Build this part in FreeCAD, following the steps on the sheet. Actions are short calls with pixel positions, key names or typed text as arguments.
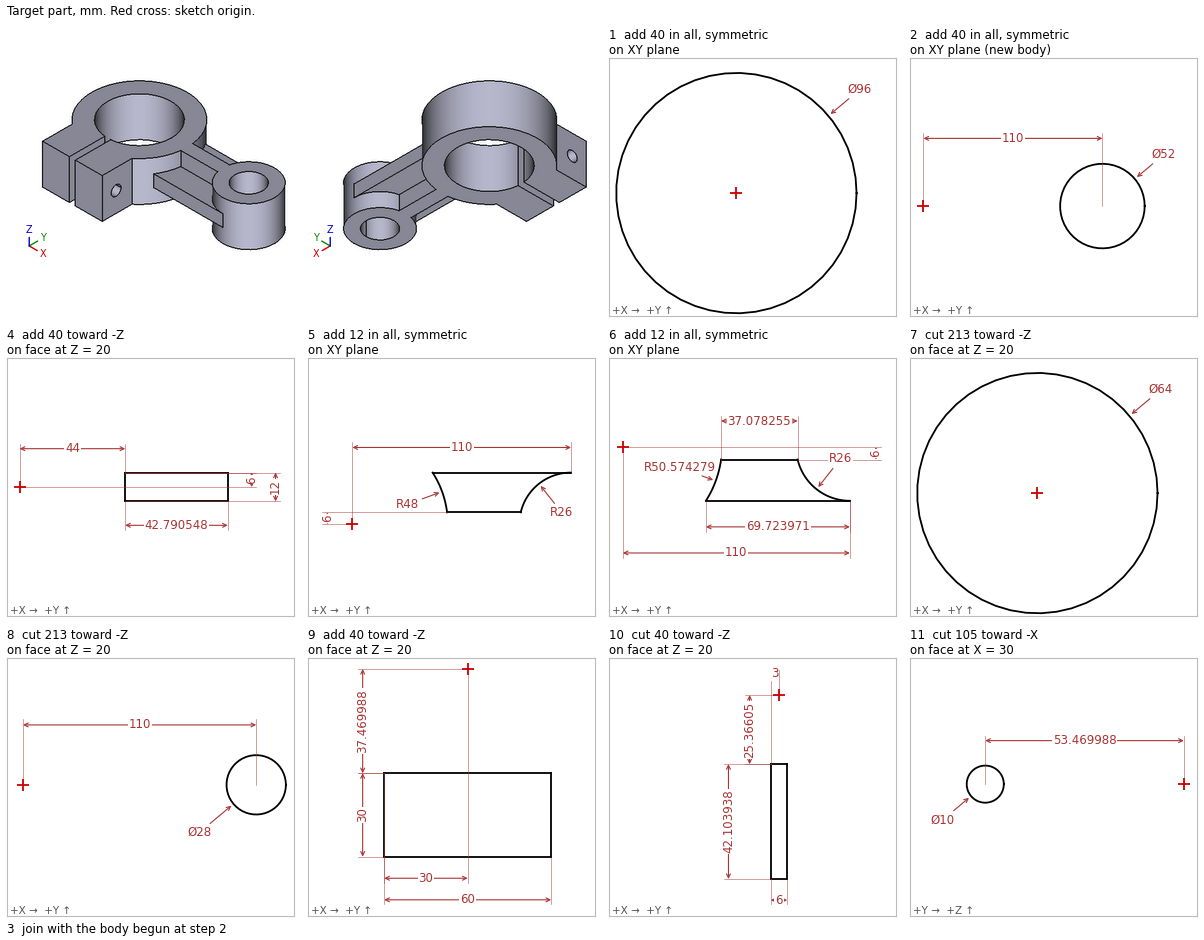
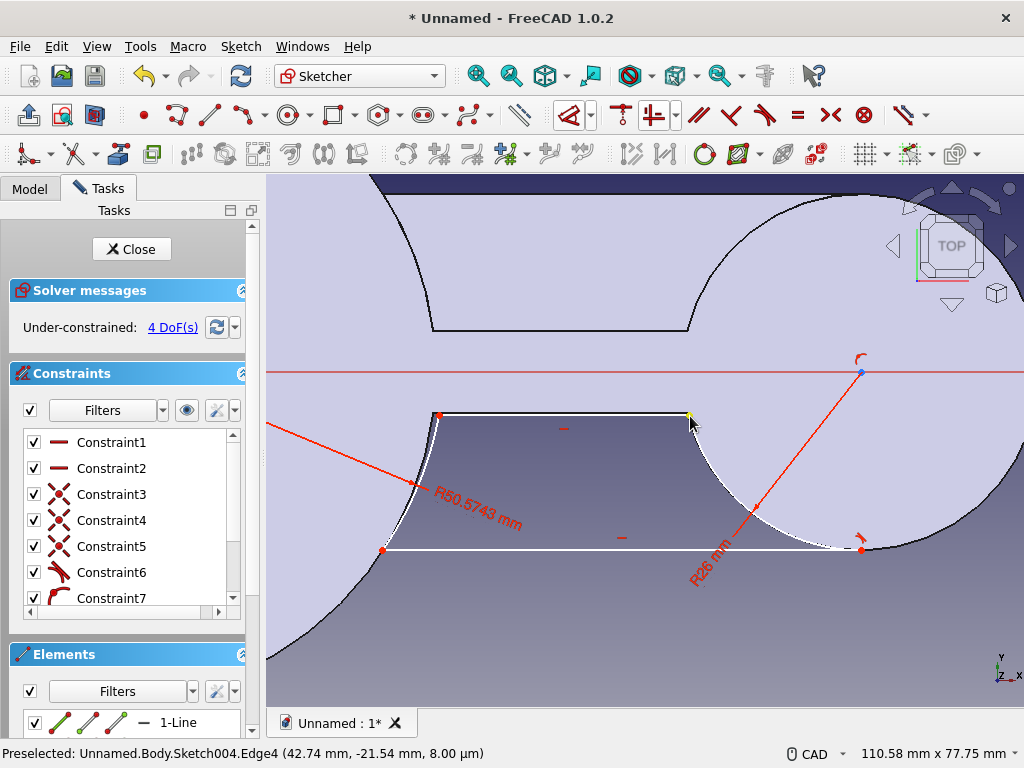
click(689, 415)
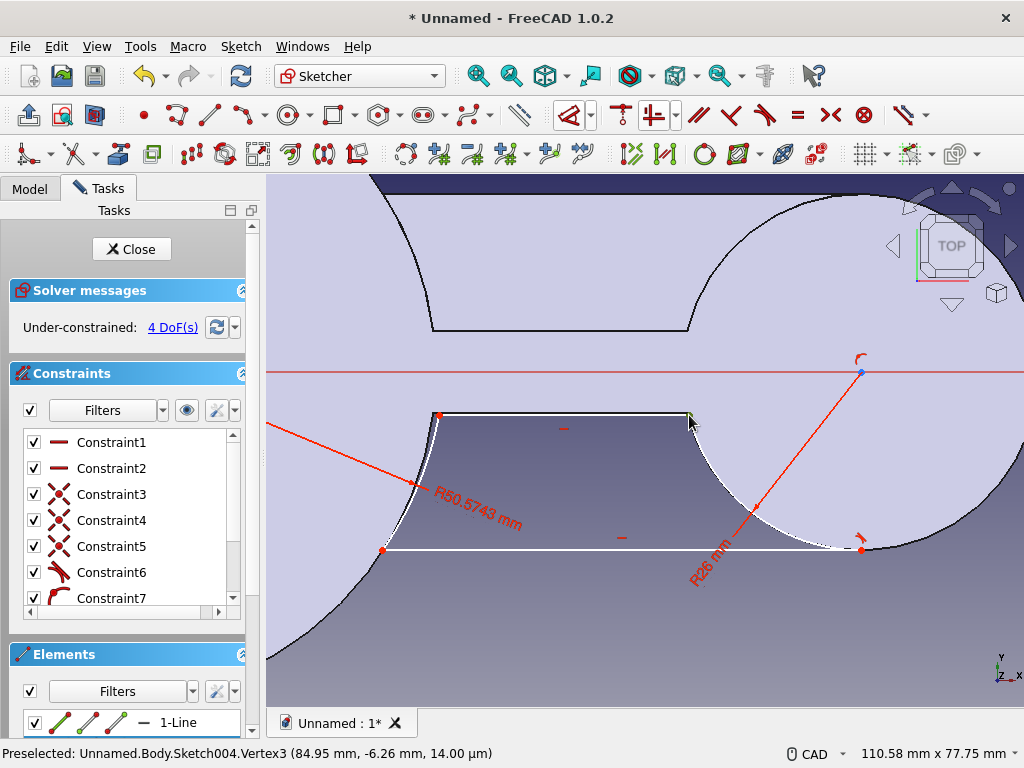
key(i)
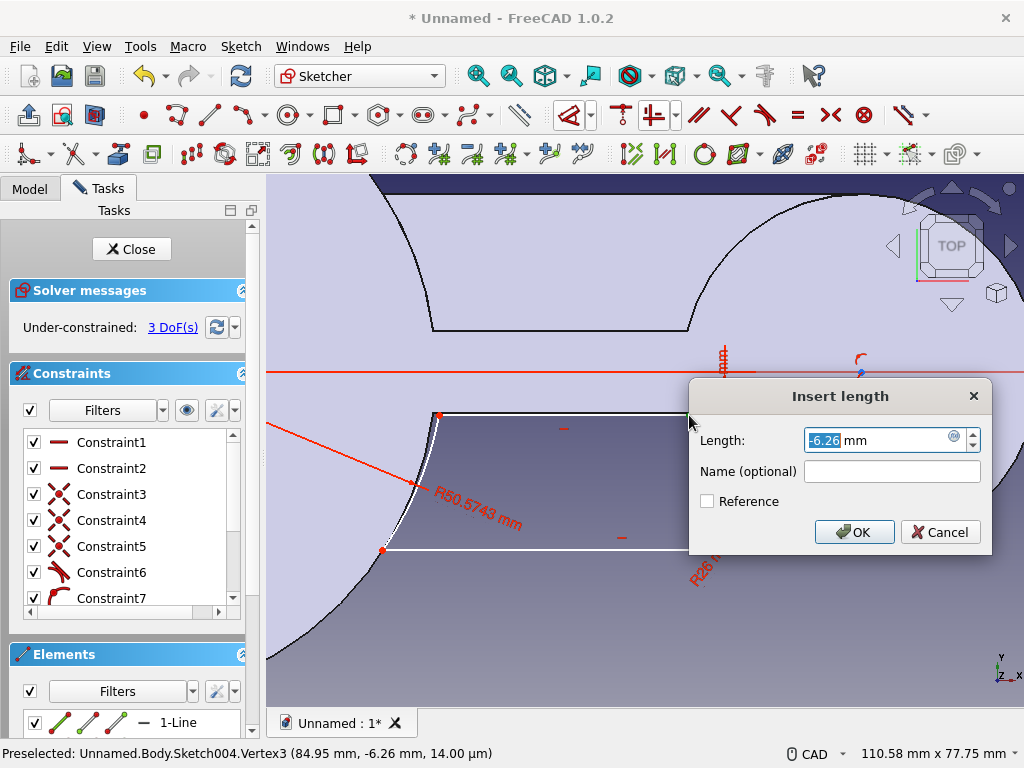
text(-6)
key(Return)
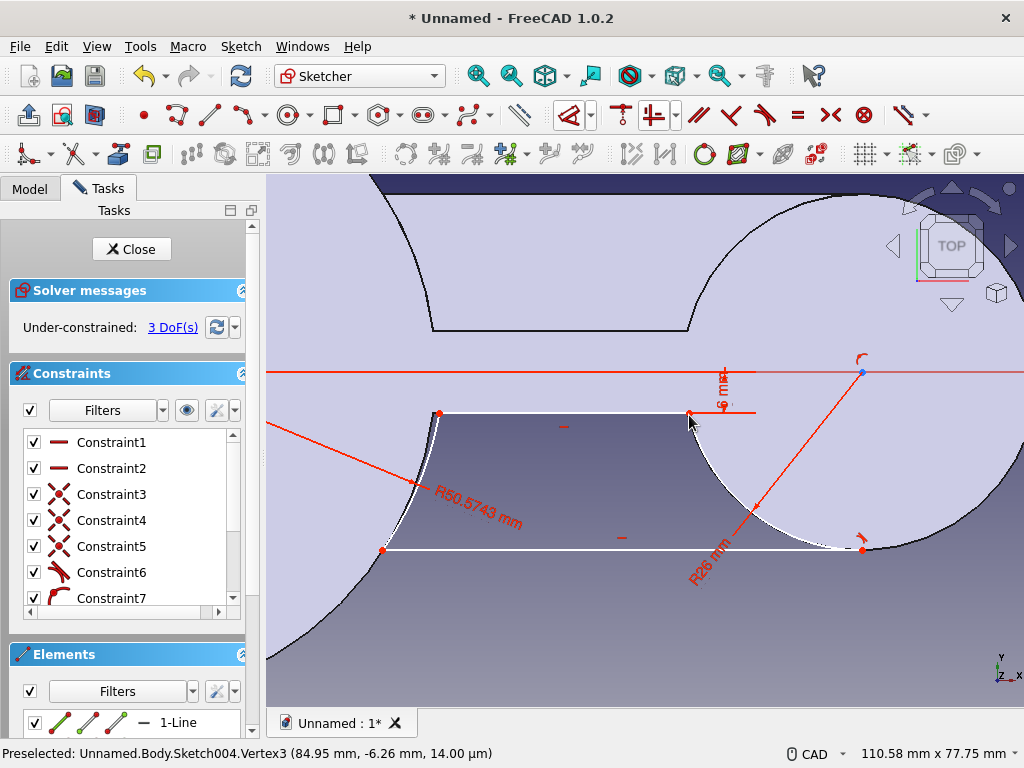
scroll(689, 415, down, 3)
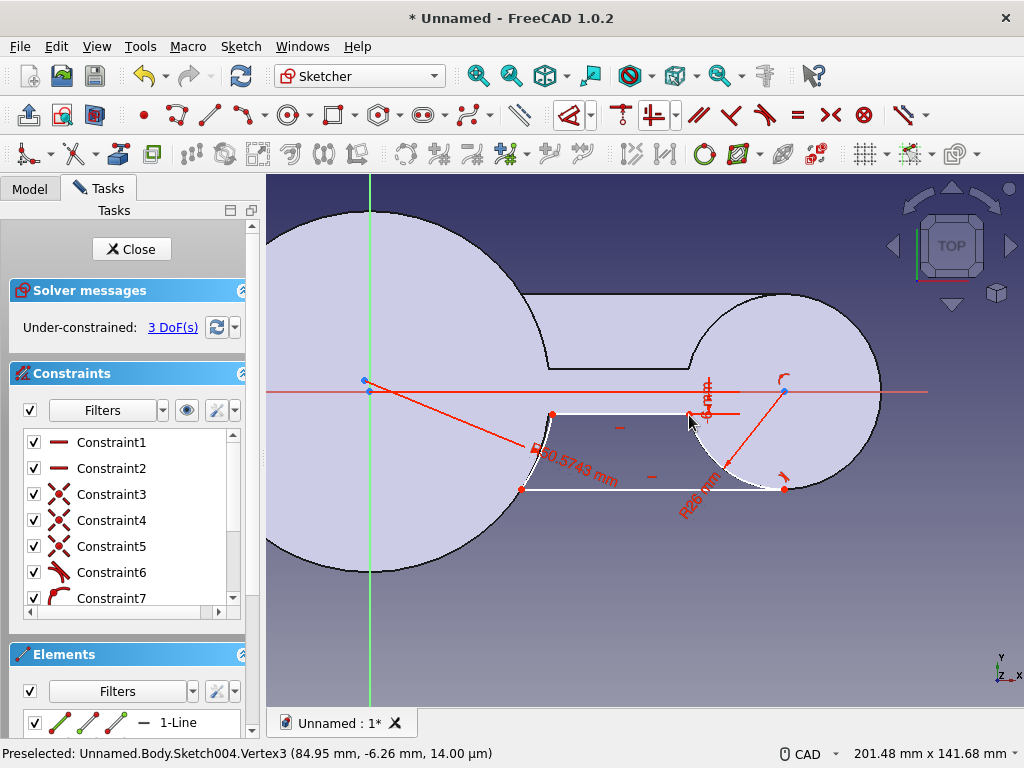
click(784, 490)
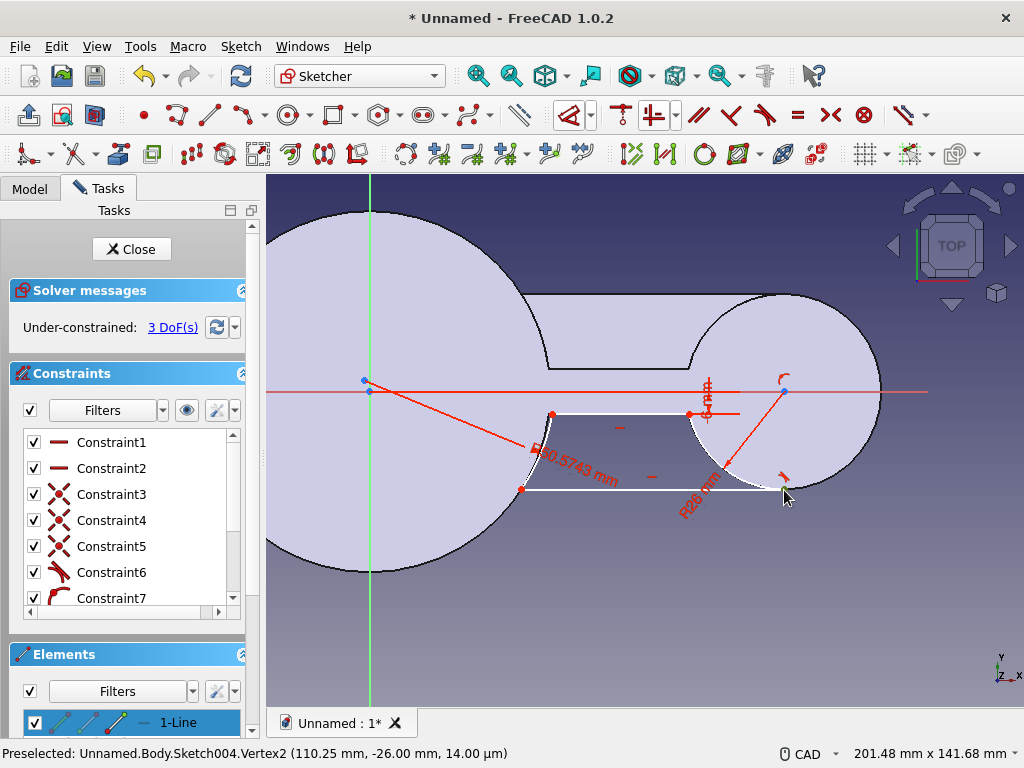
key(l)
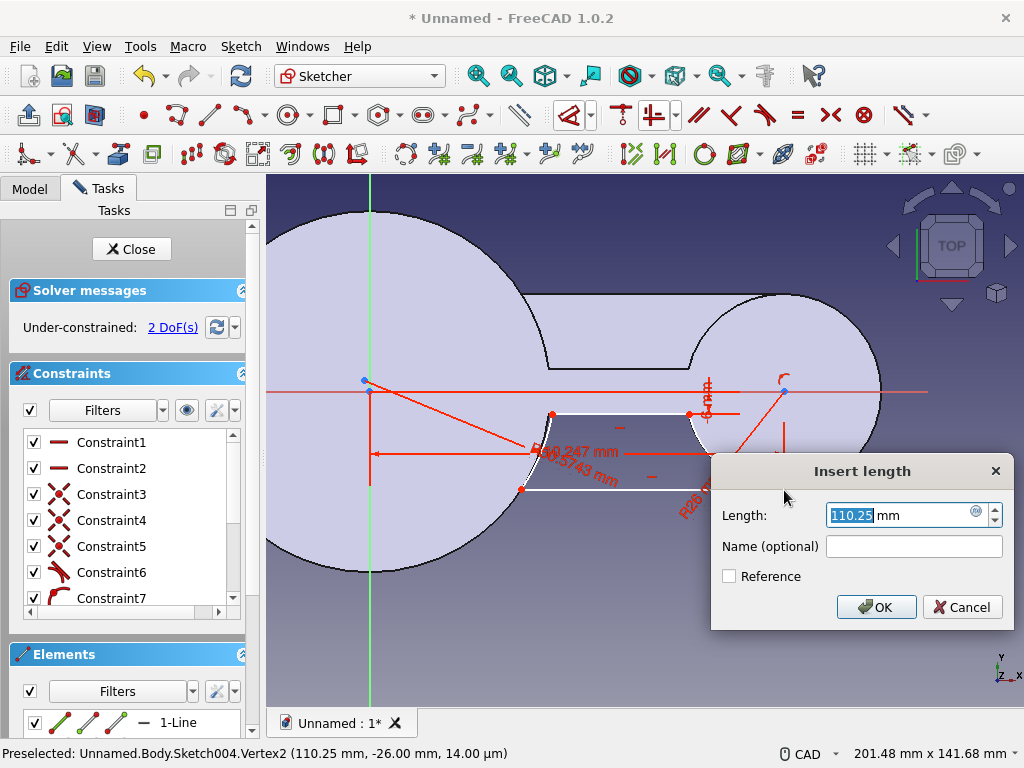
text(110)
key(Return)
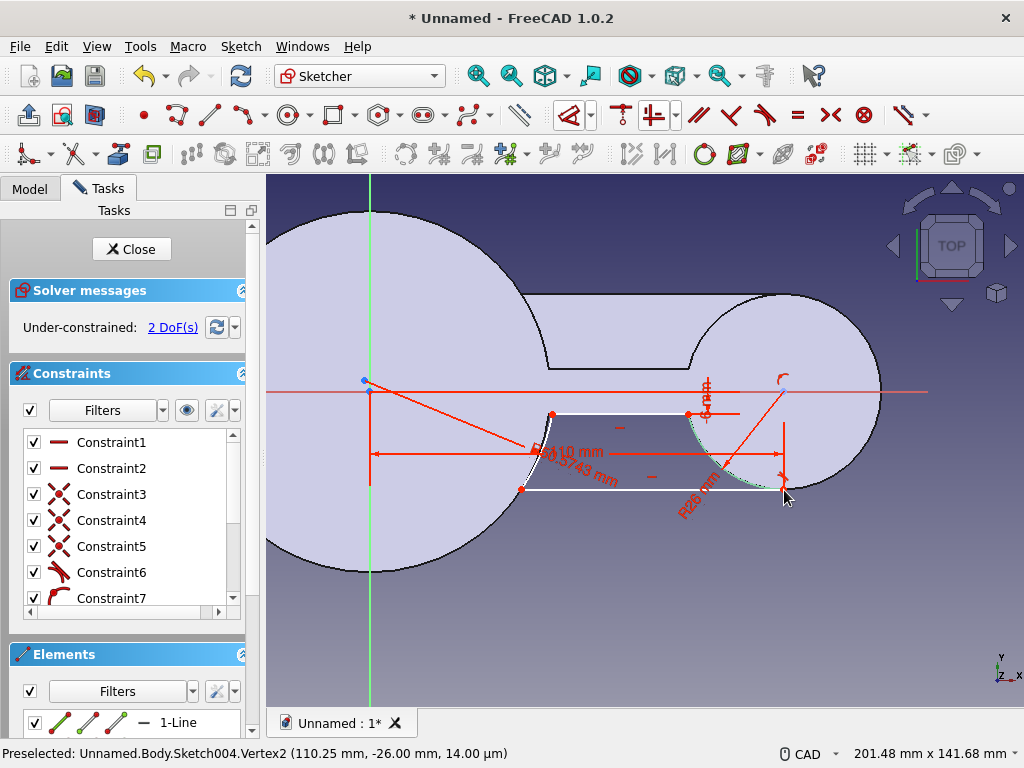
click(600, 490)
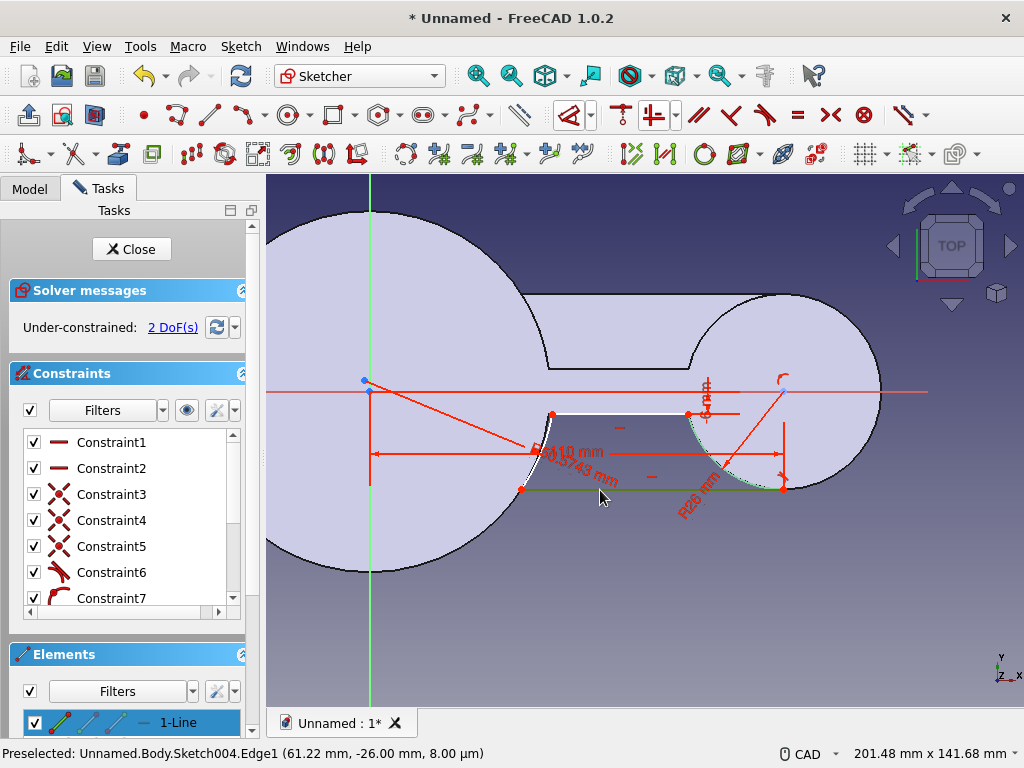
click(590, 116)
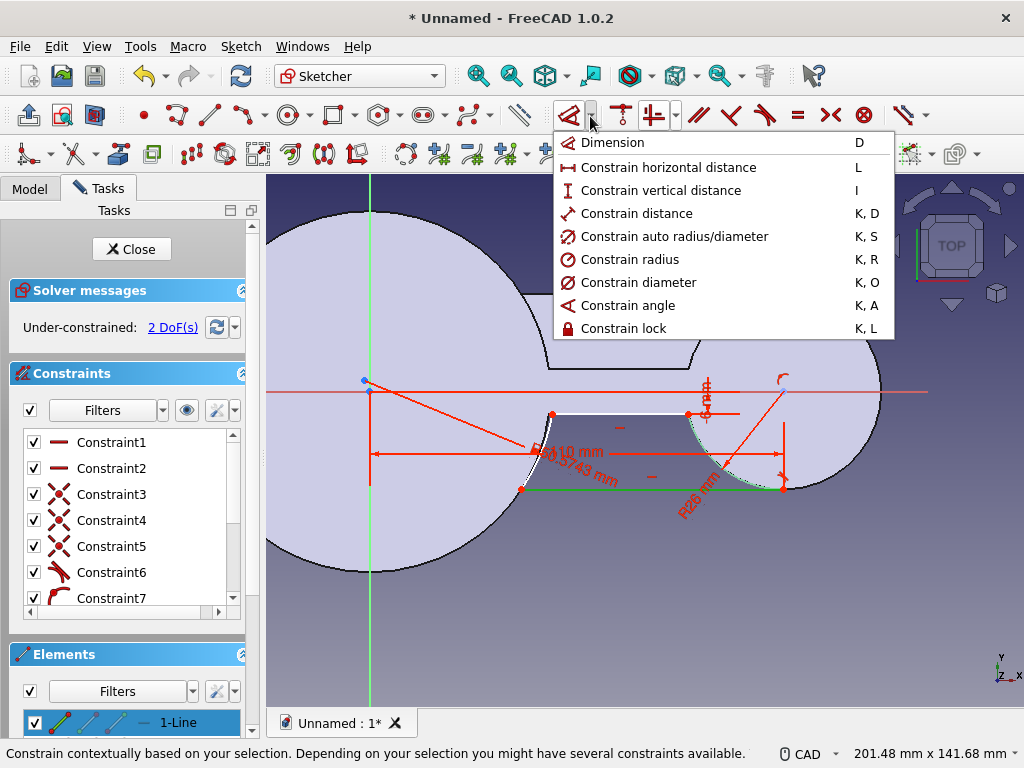
click(724, 168)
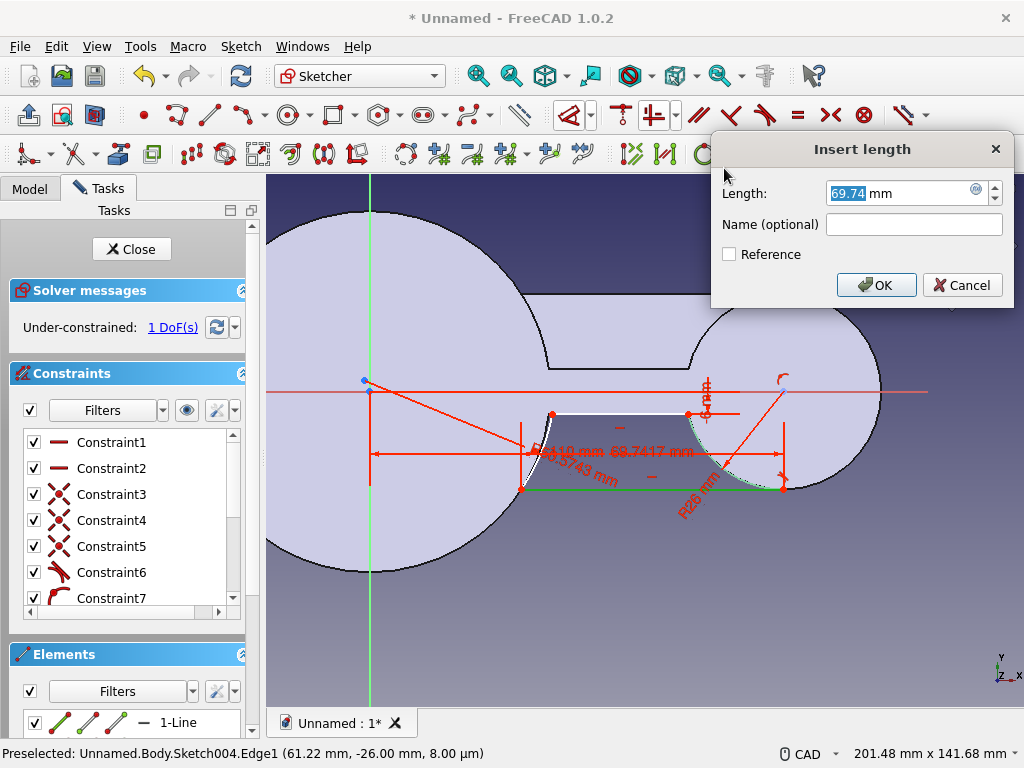
text(69.723971)
key(Return)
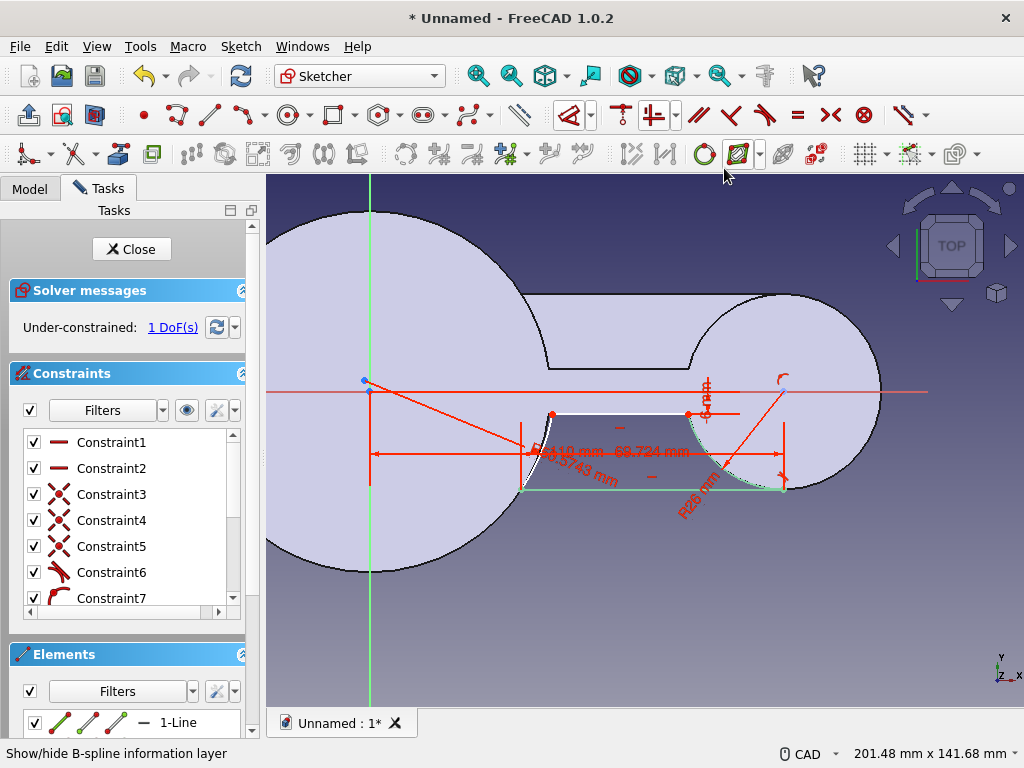
click(648, 414)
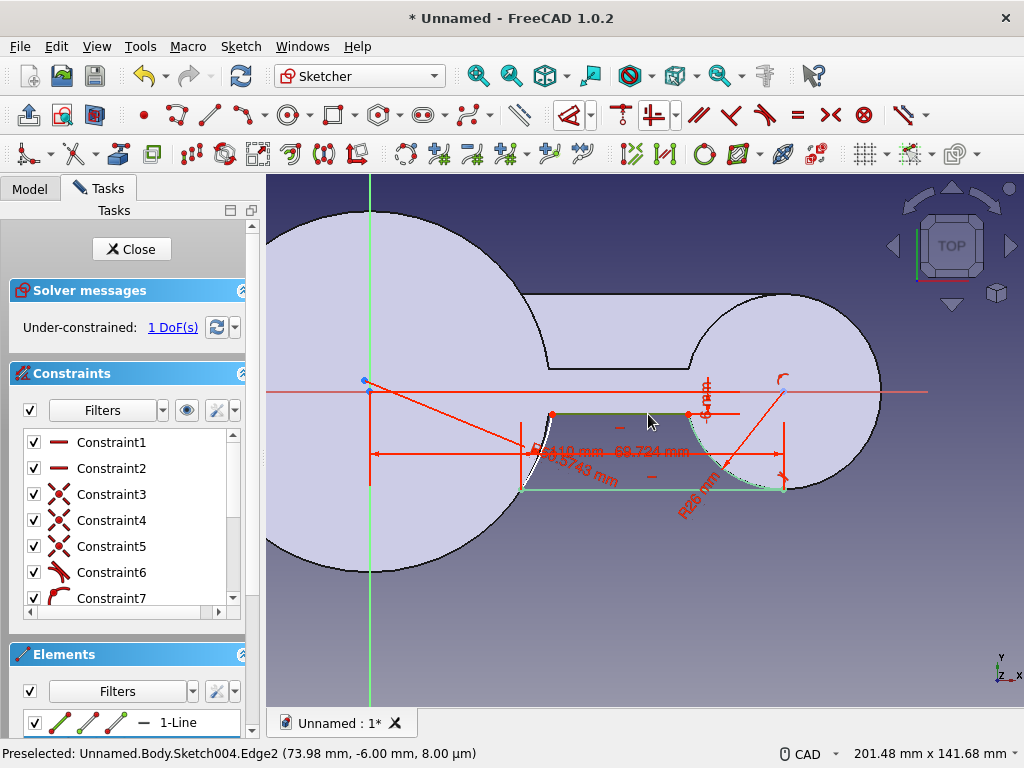
click(590, 116)